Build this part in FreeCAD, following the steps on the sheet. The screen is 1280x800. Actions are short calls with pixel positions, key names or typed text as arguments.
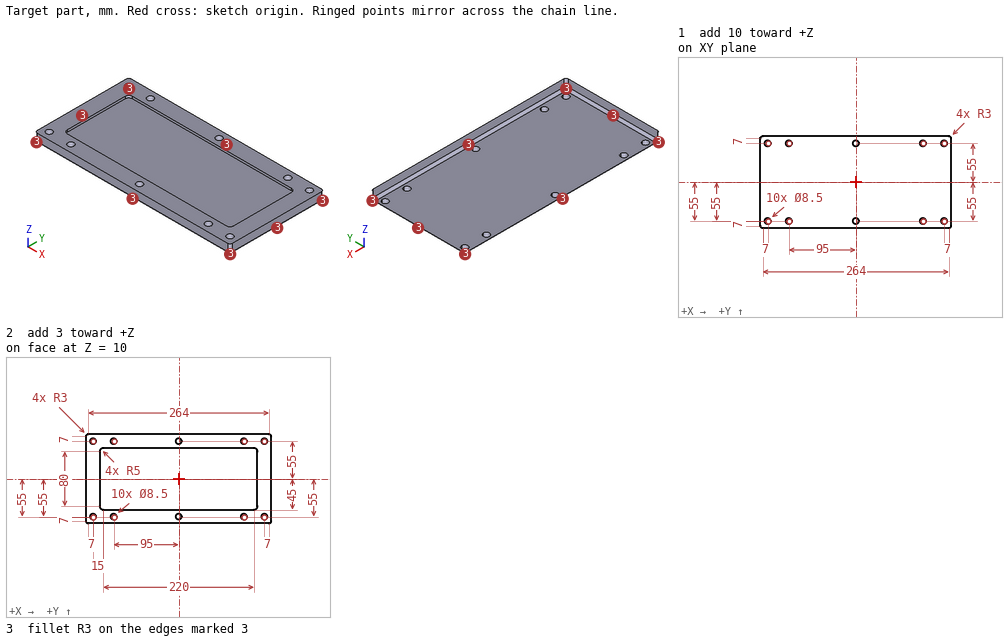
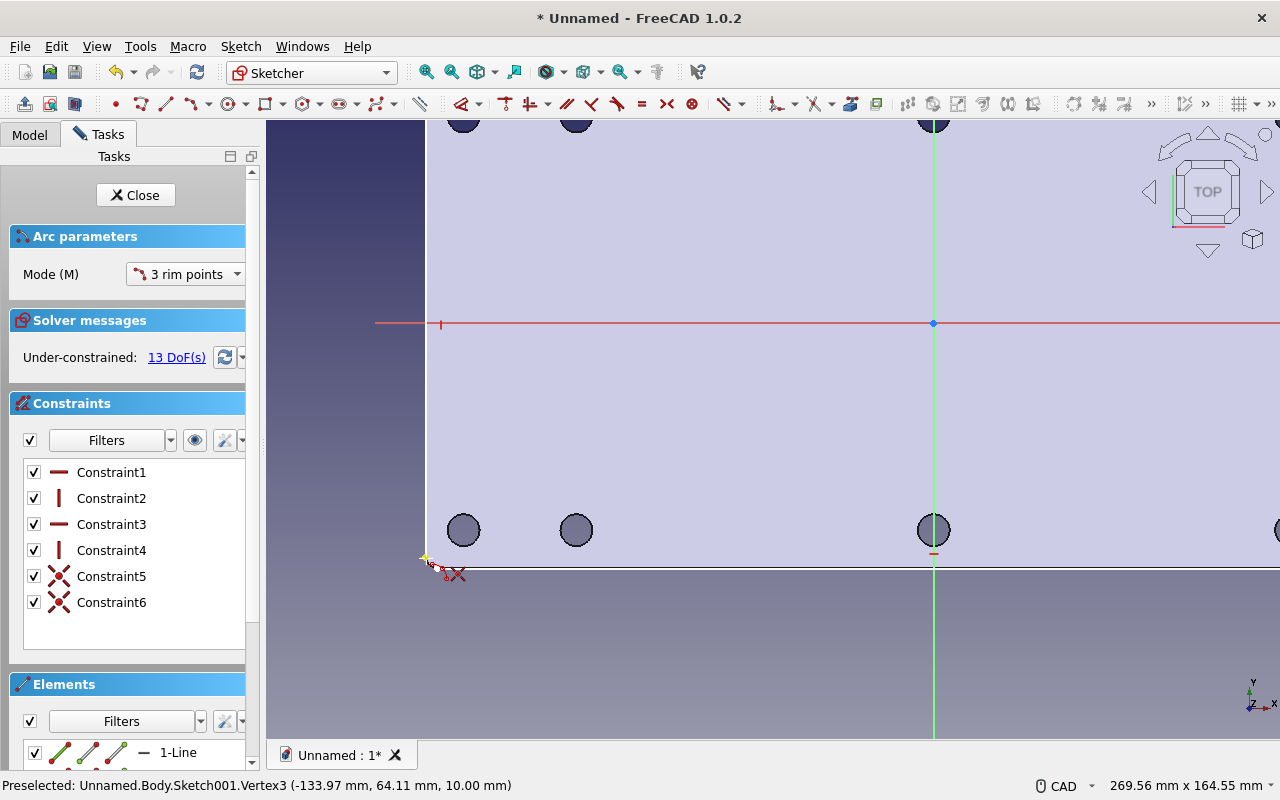
click(426, 557)
click(438, 569)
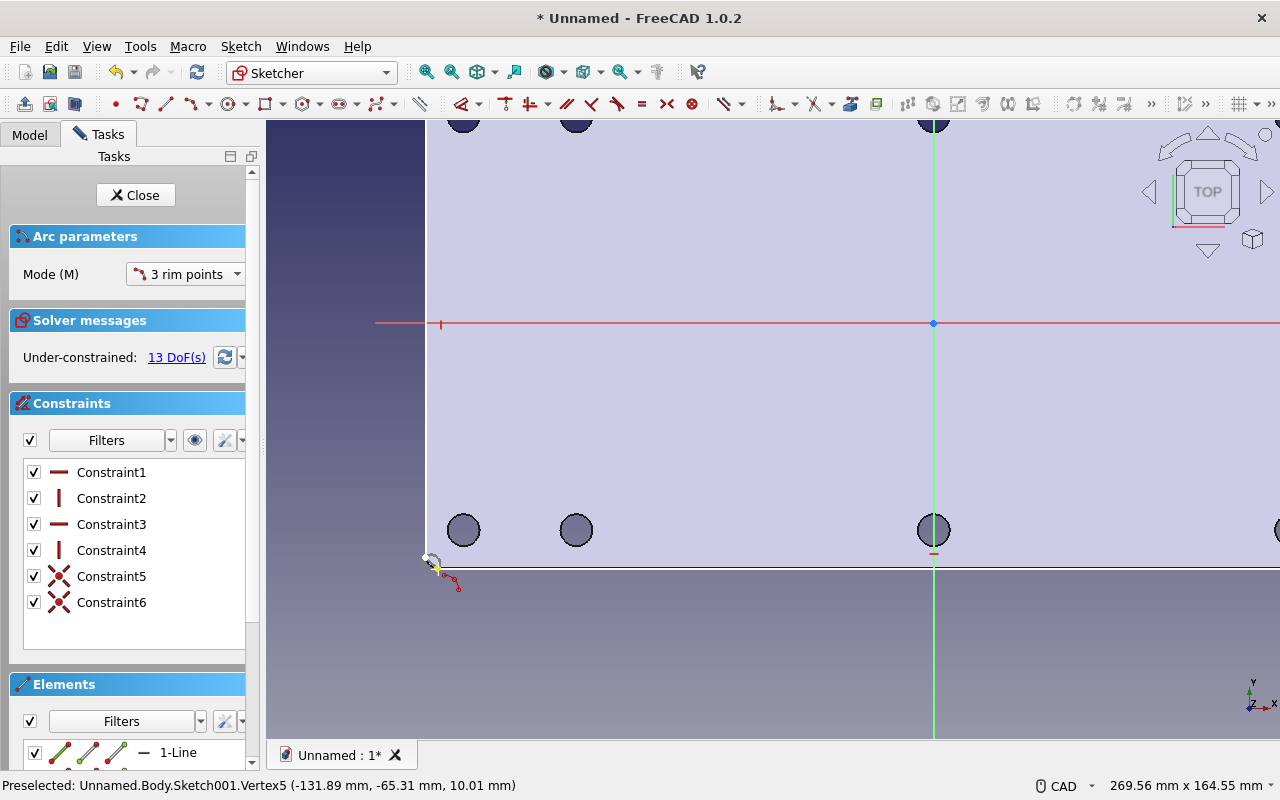
scroll(429, 565, up, 8)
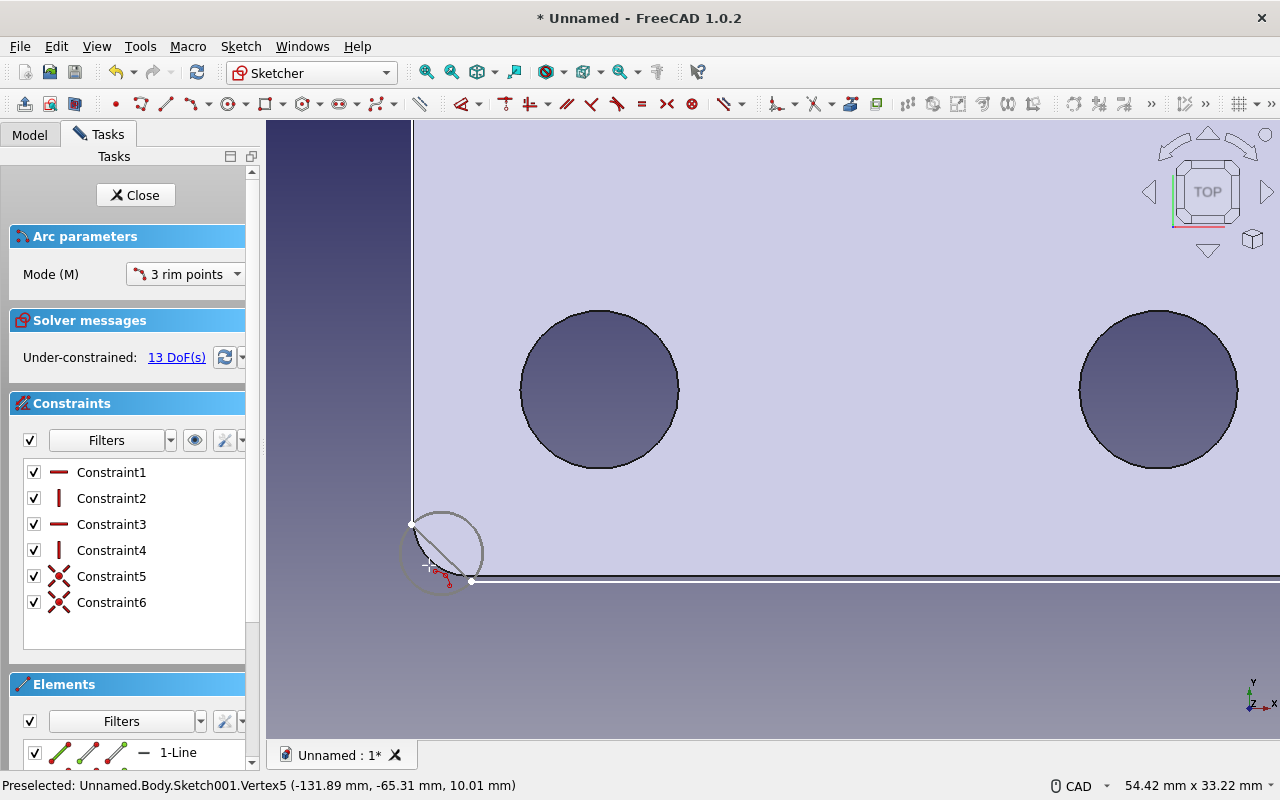
click(430, 560)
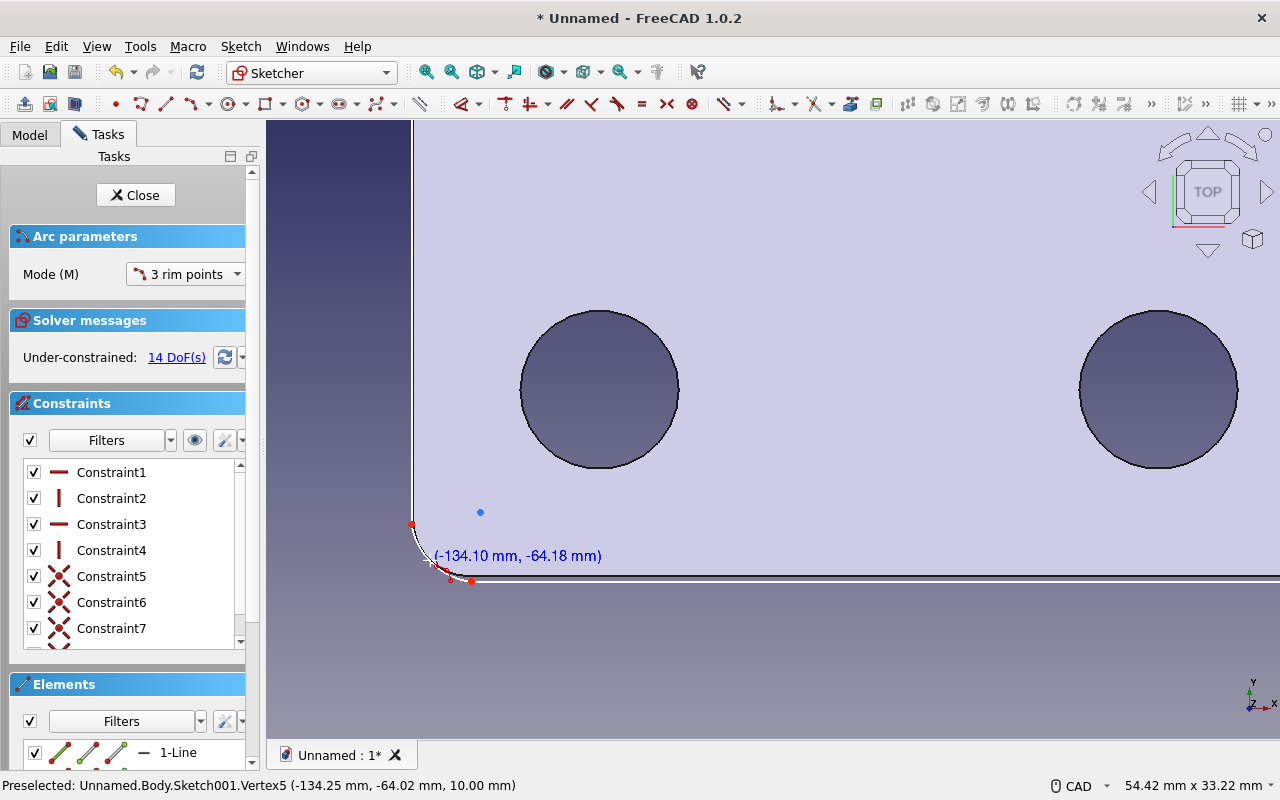
scroll(427, 562, down, 11)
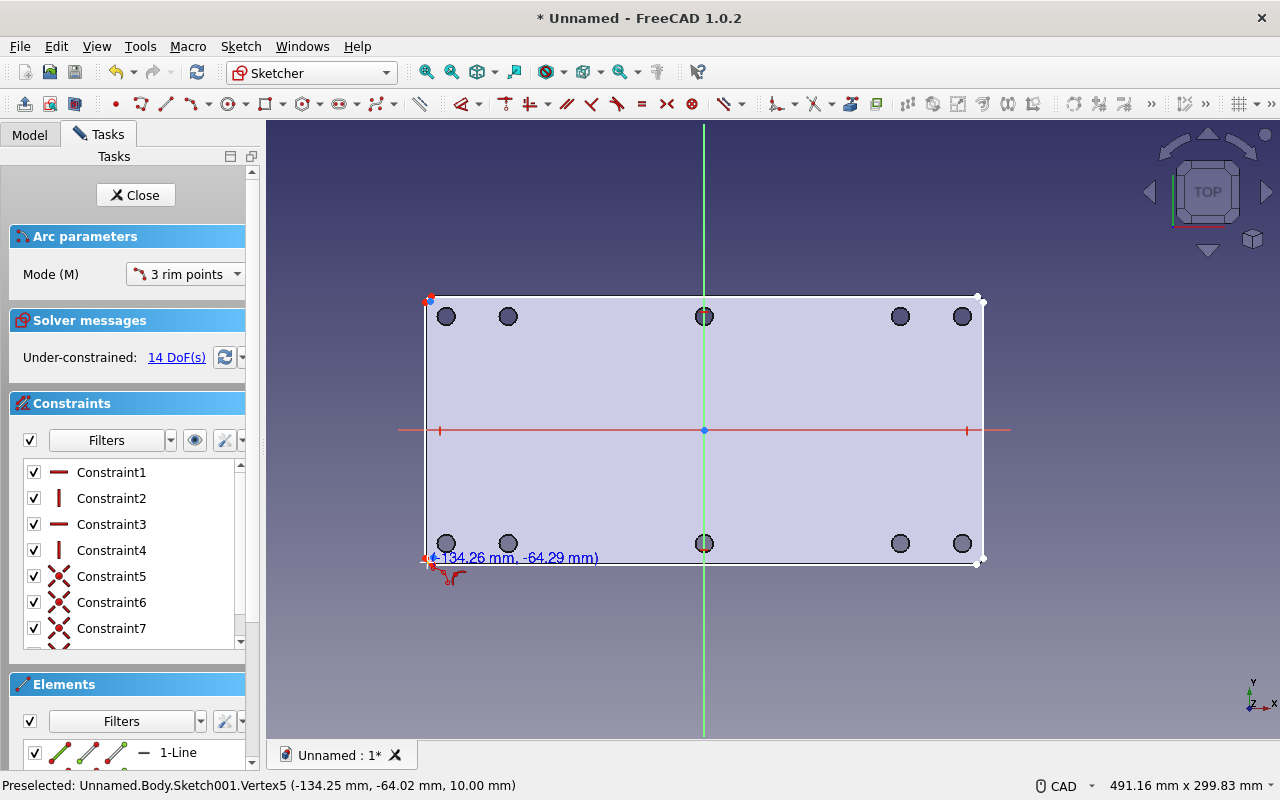
scroll(977, 564, up, 3)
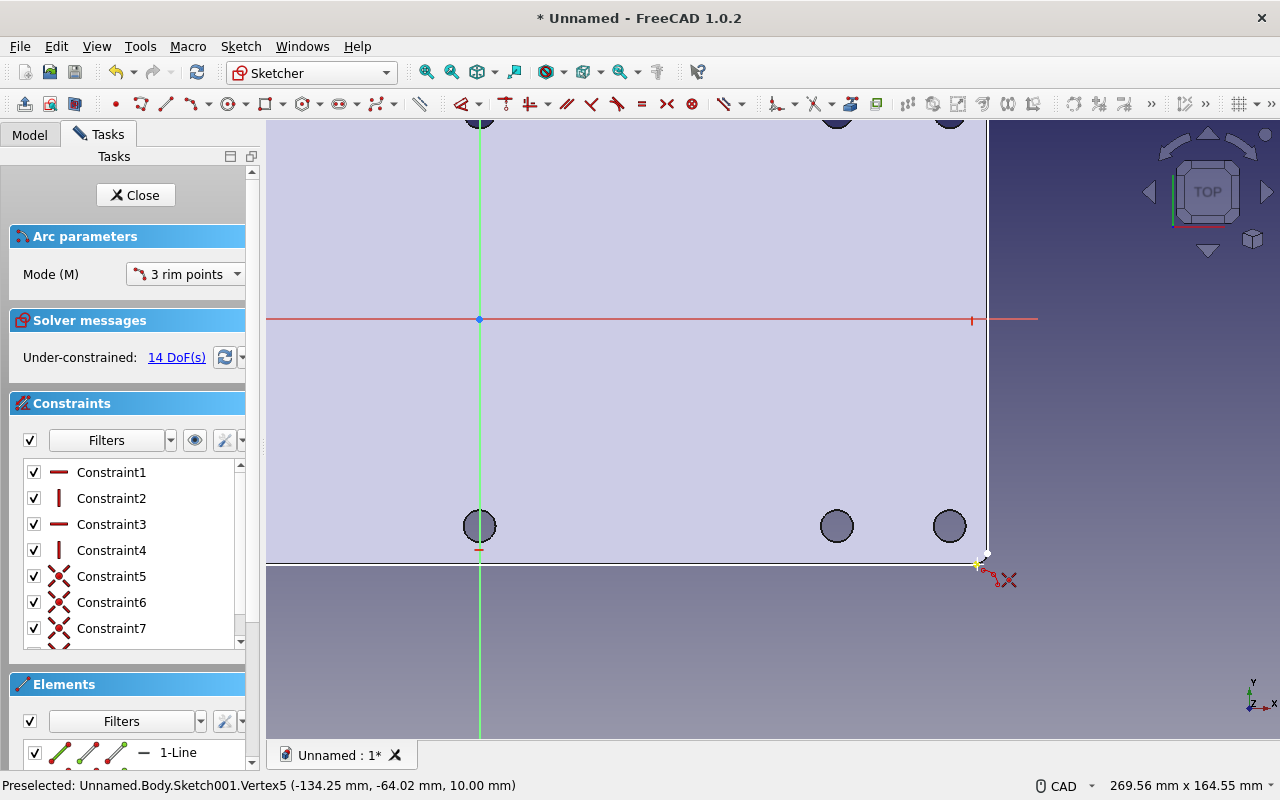
click(976, 565)
click(988, 553)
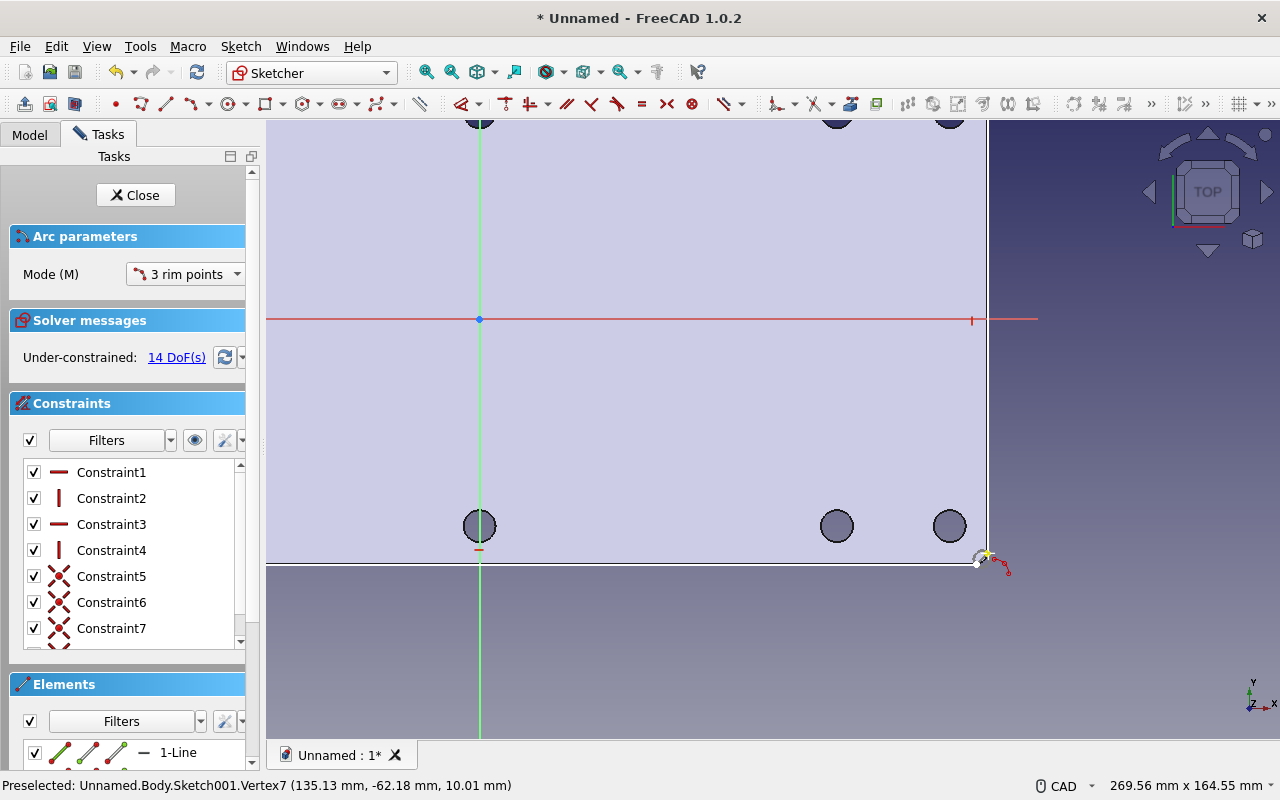
scroll(984, 560, up, 8)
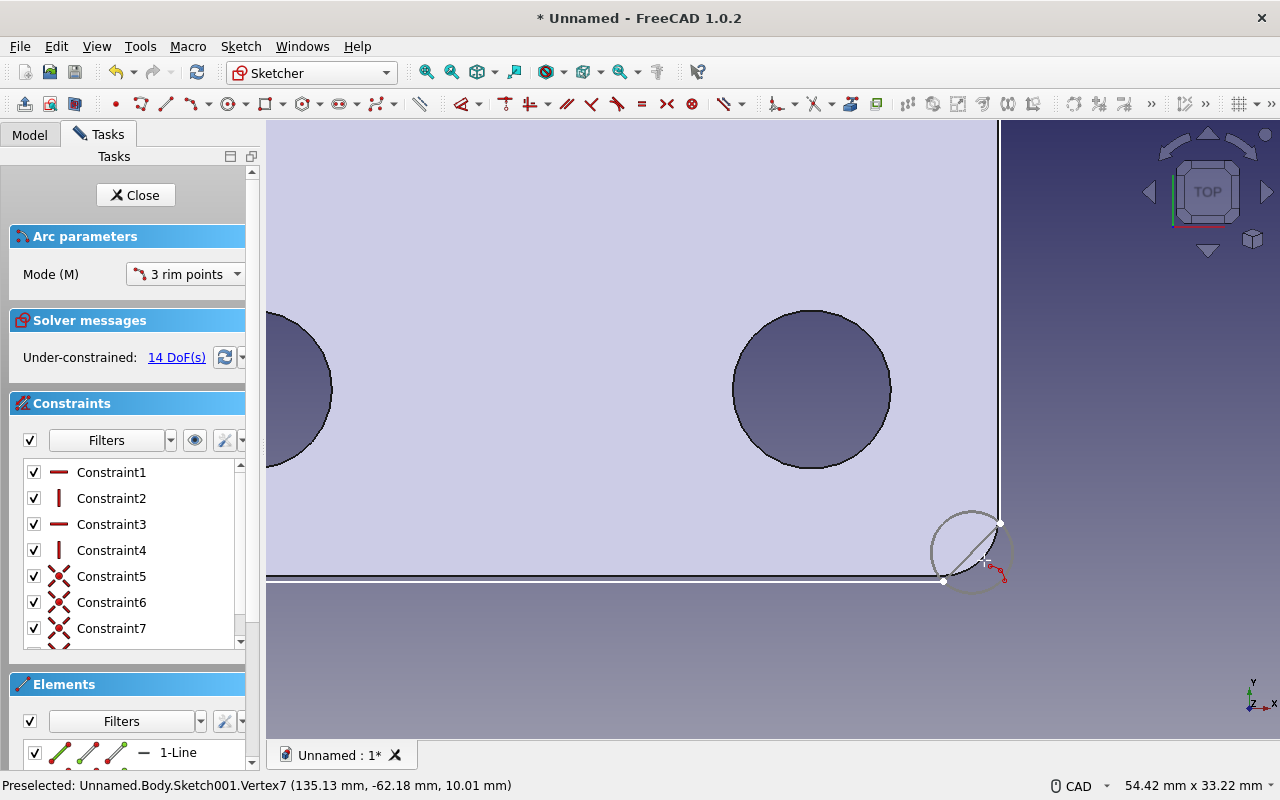
click(982, 560)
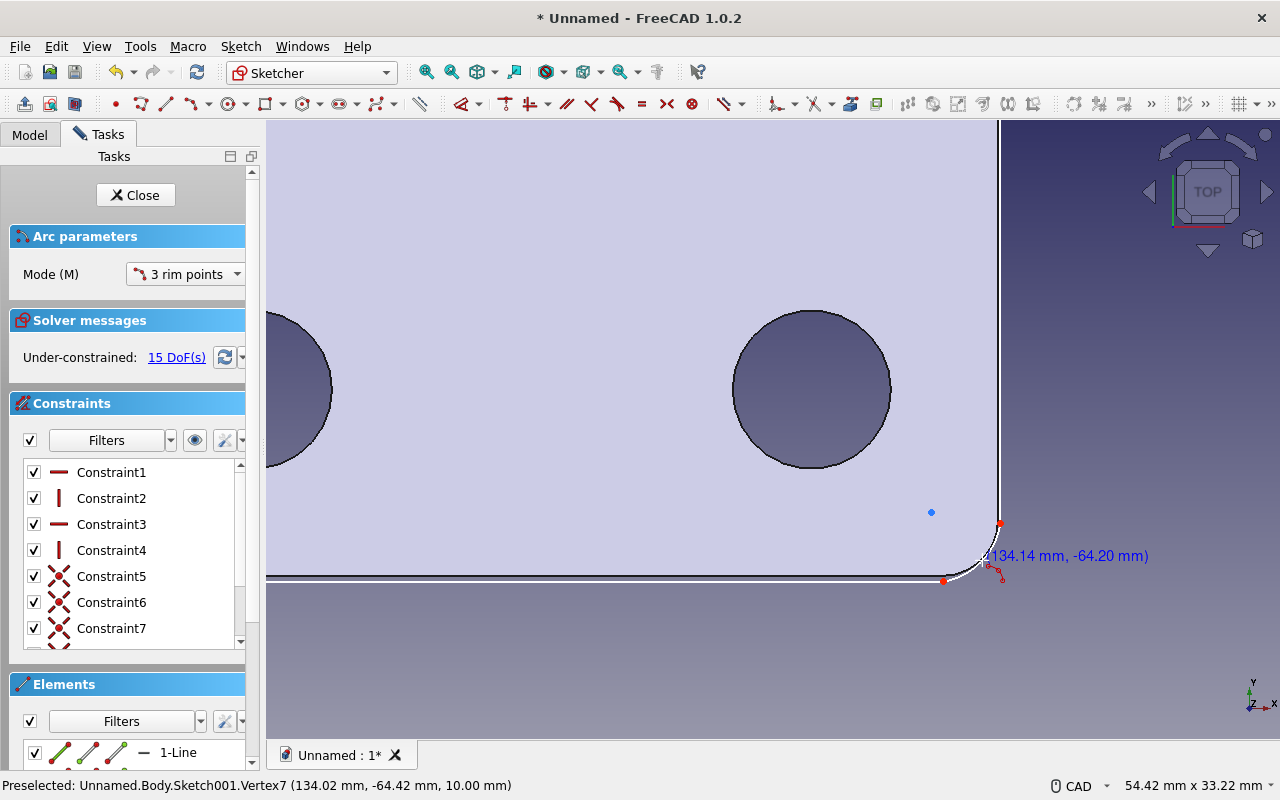
scroll(981, 562, down, 11)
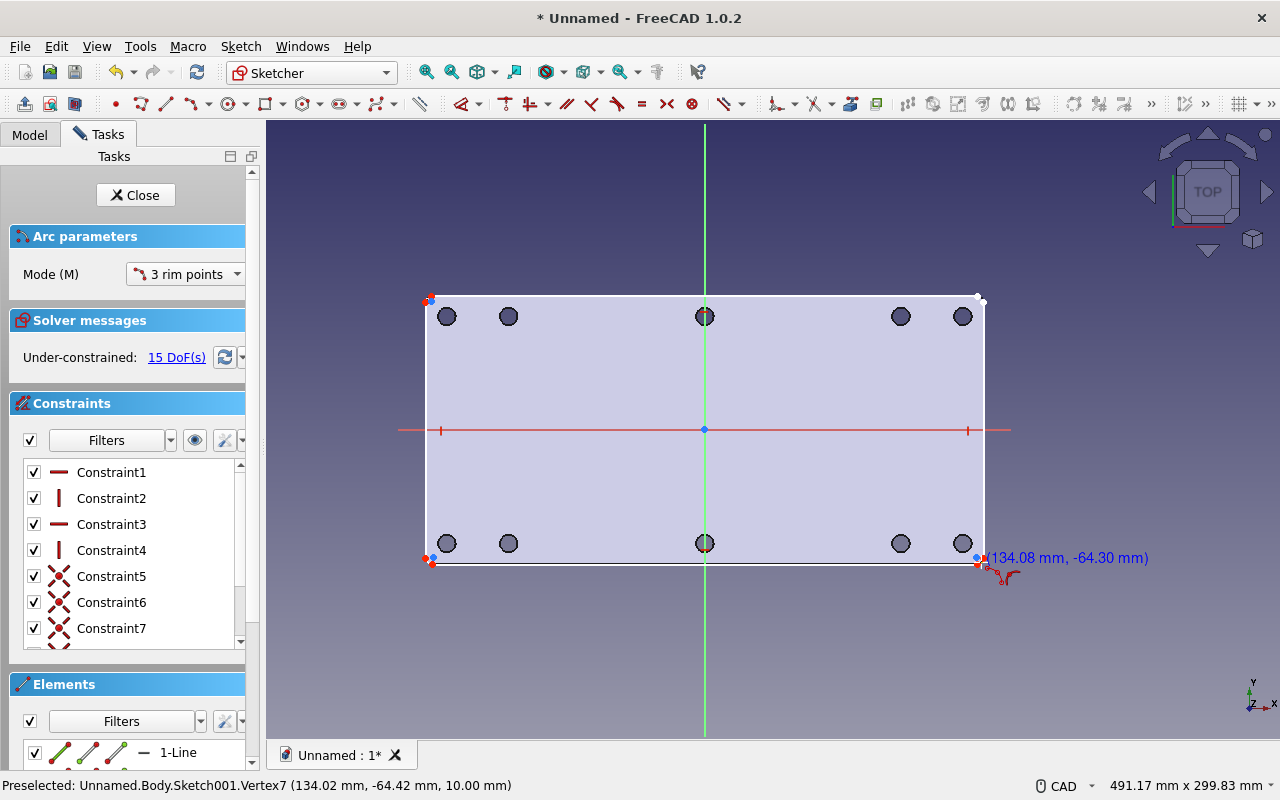
scroll(984, 302, up, 3)